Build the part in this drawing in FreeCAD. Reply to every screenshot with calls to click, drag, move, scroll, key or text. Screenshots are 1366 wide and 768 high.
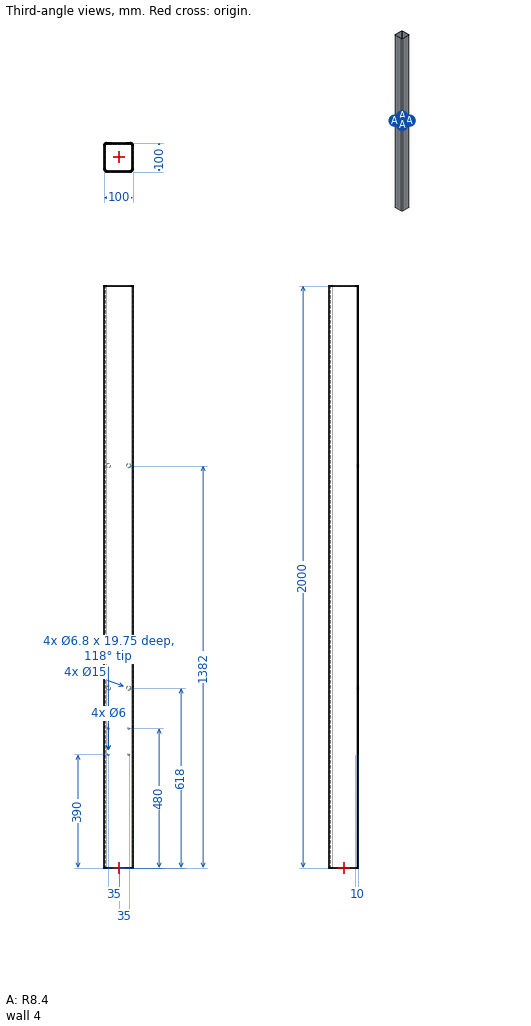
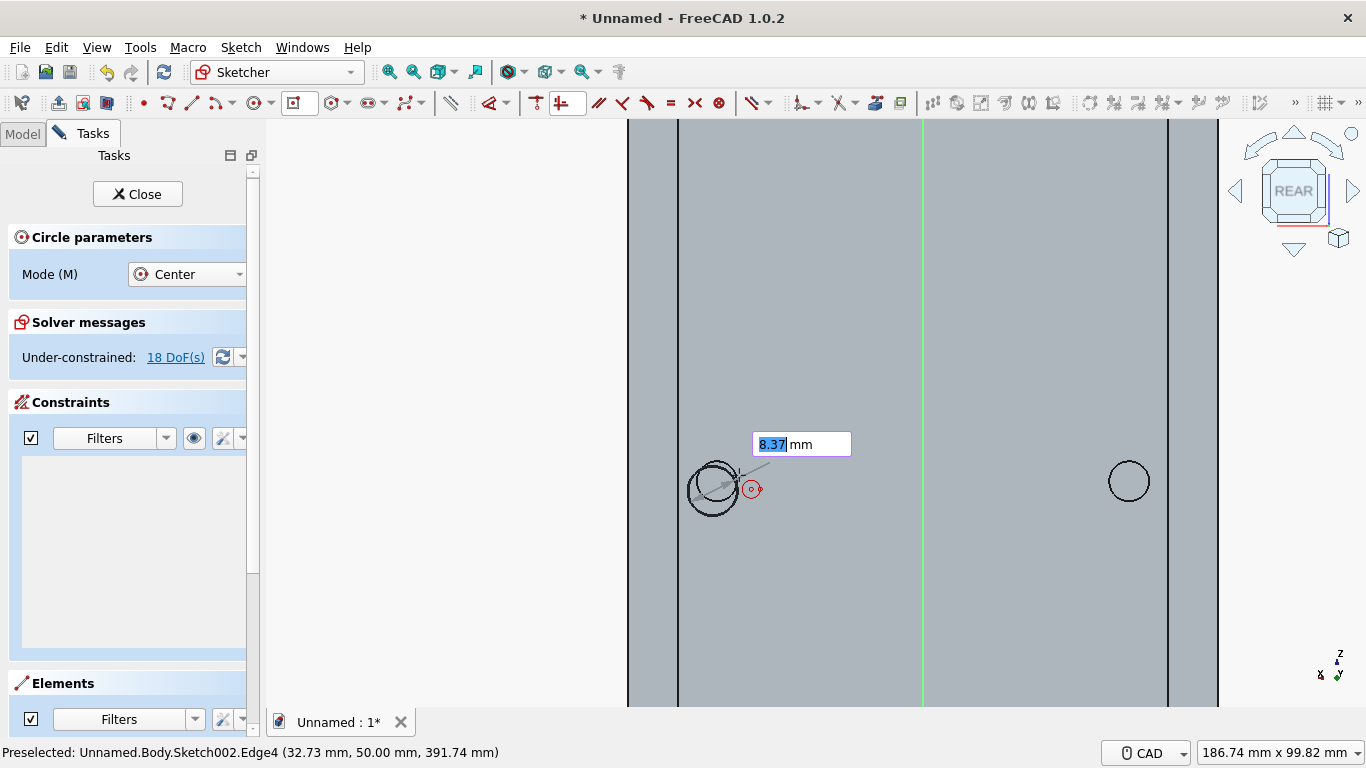
click(729, 469)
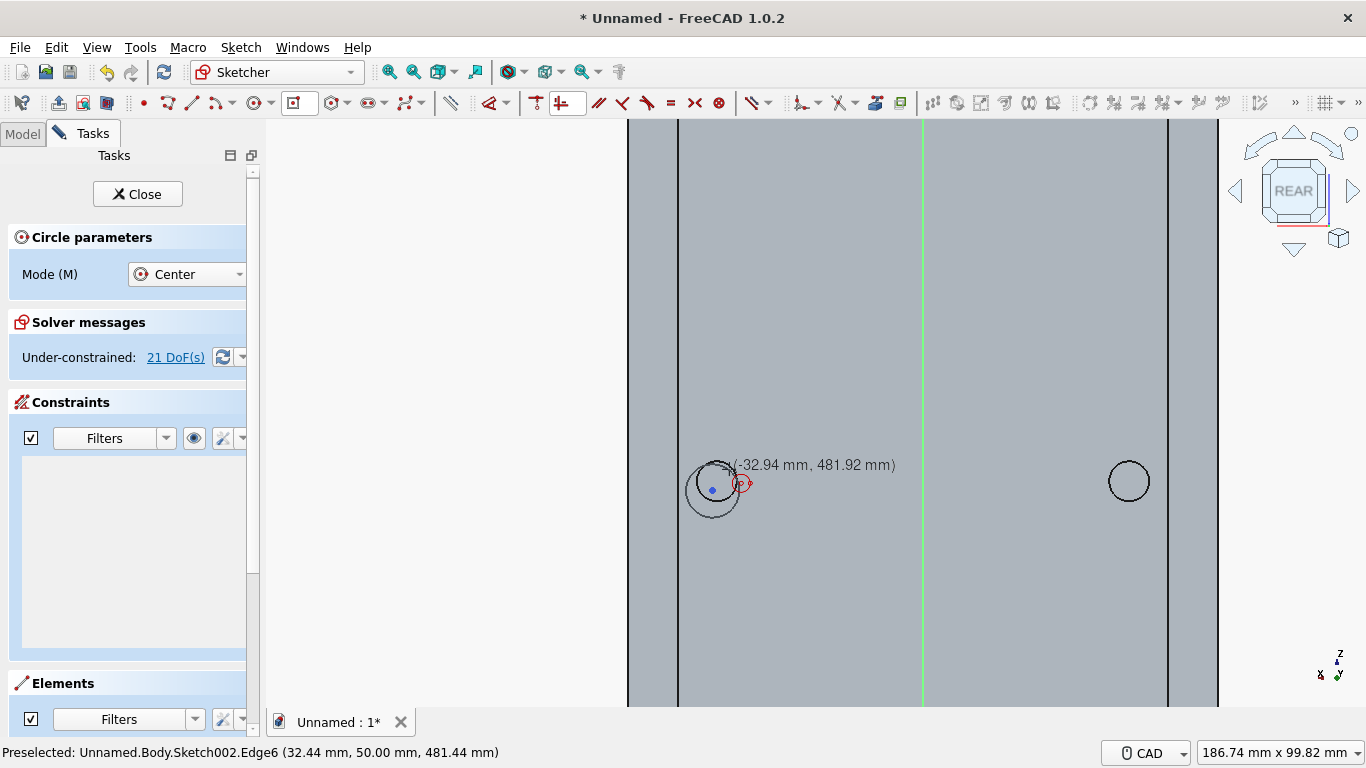
scroll(1129, 481, up, 2)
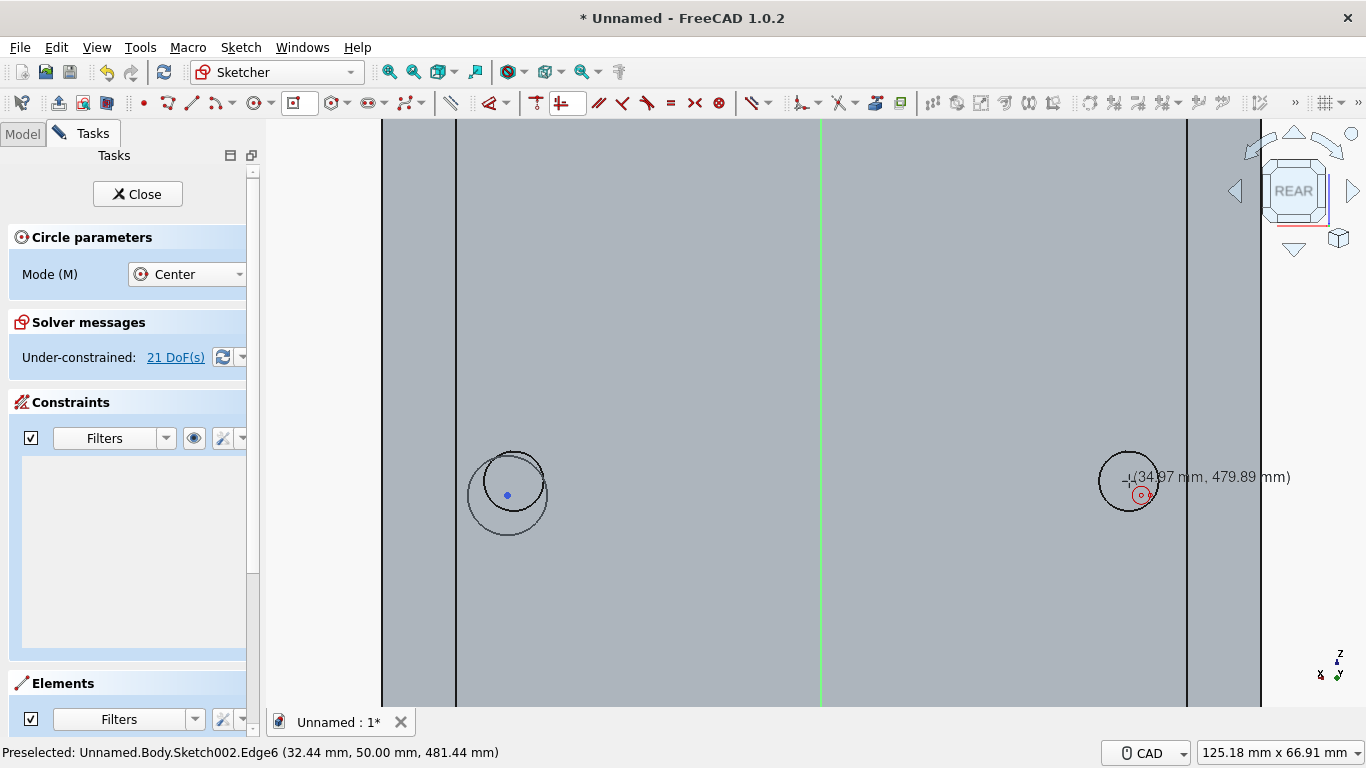
scroll(745, 476, down, 17)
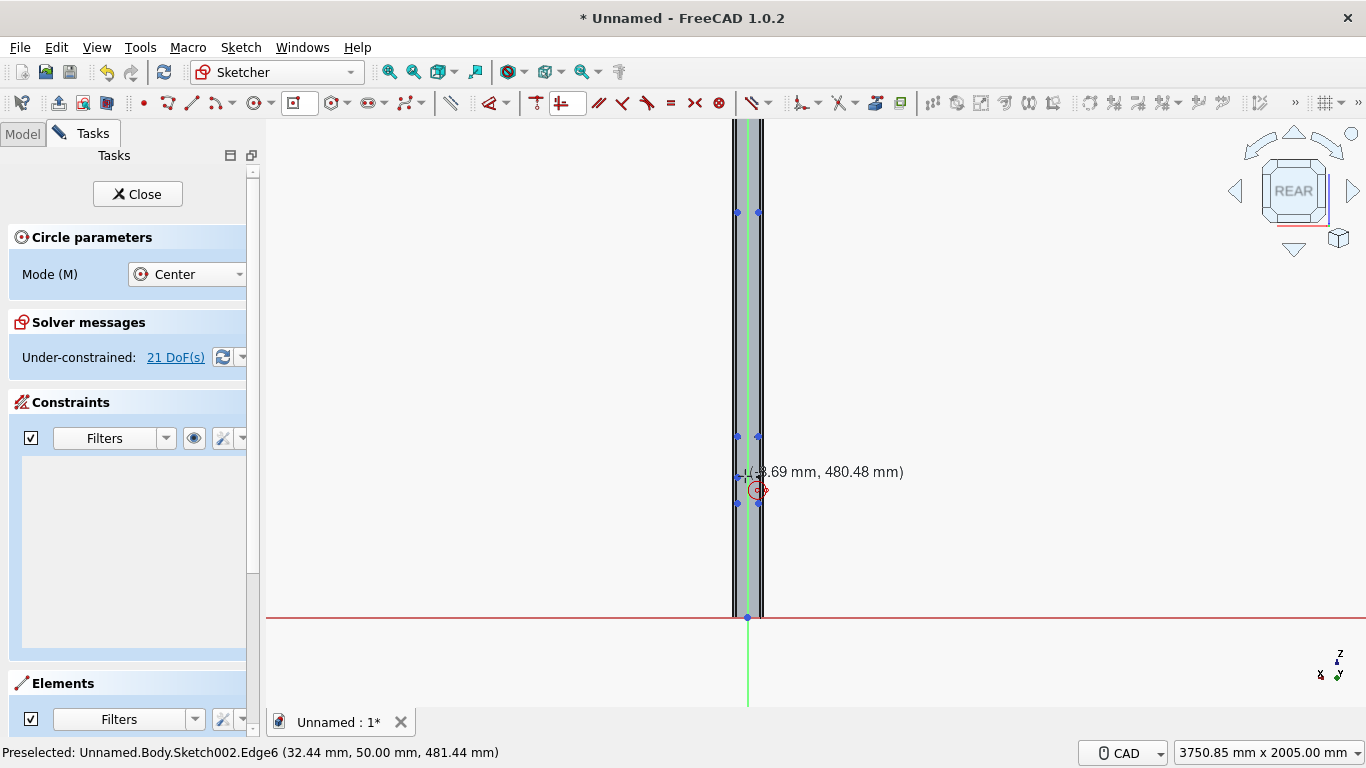
scroll(758, 477, up, 3)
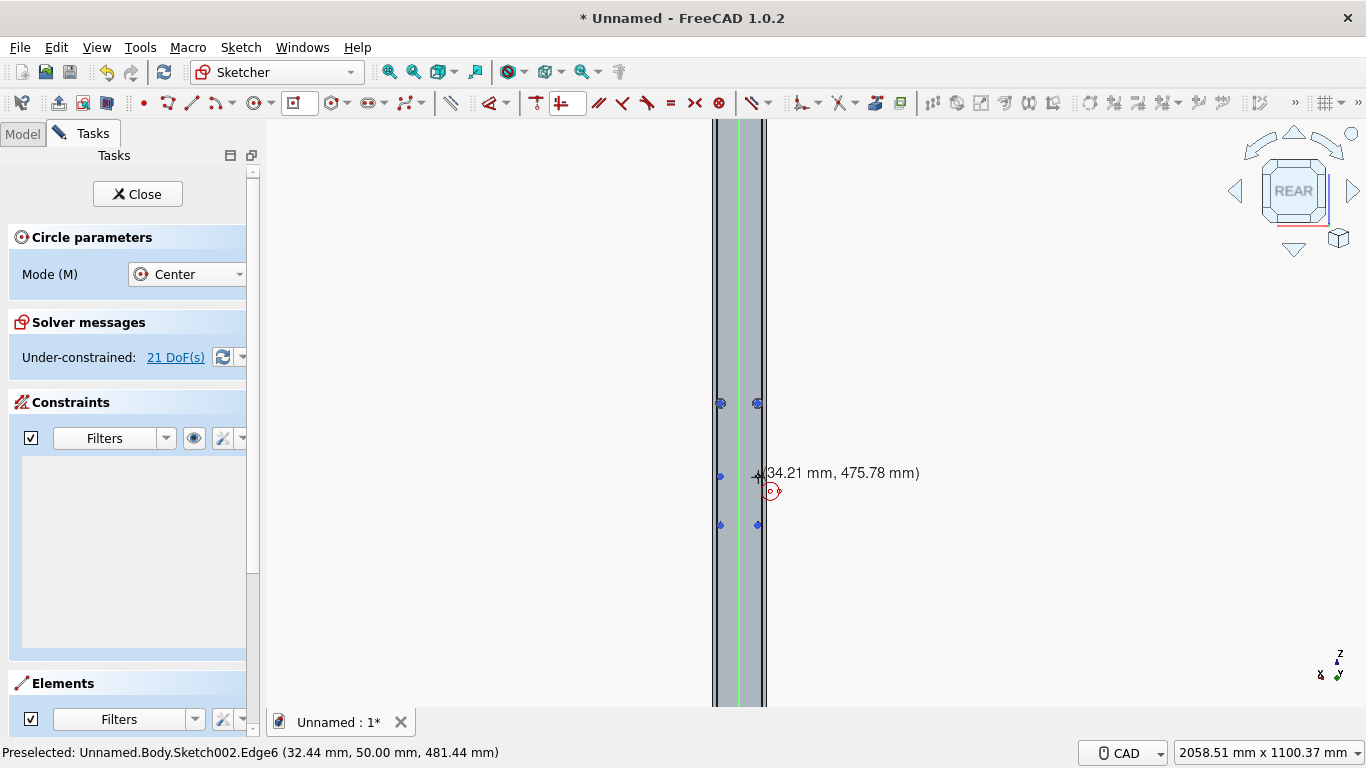
click(758, 476)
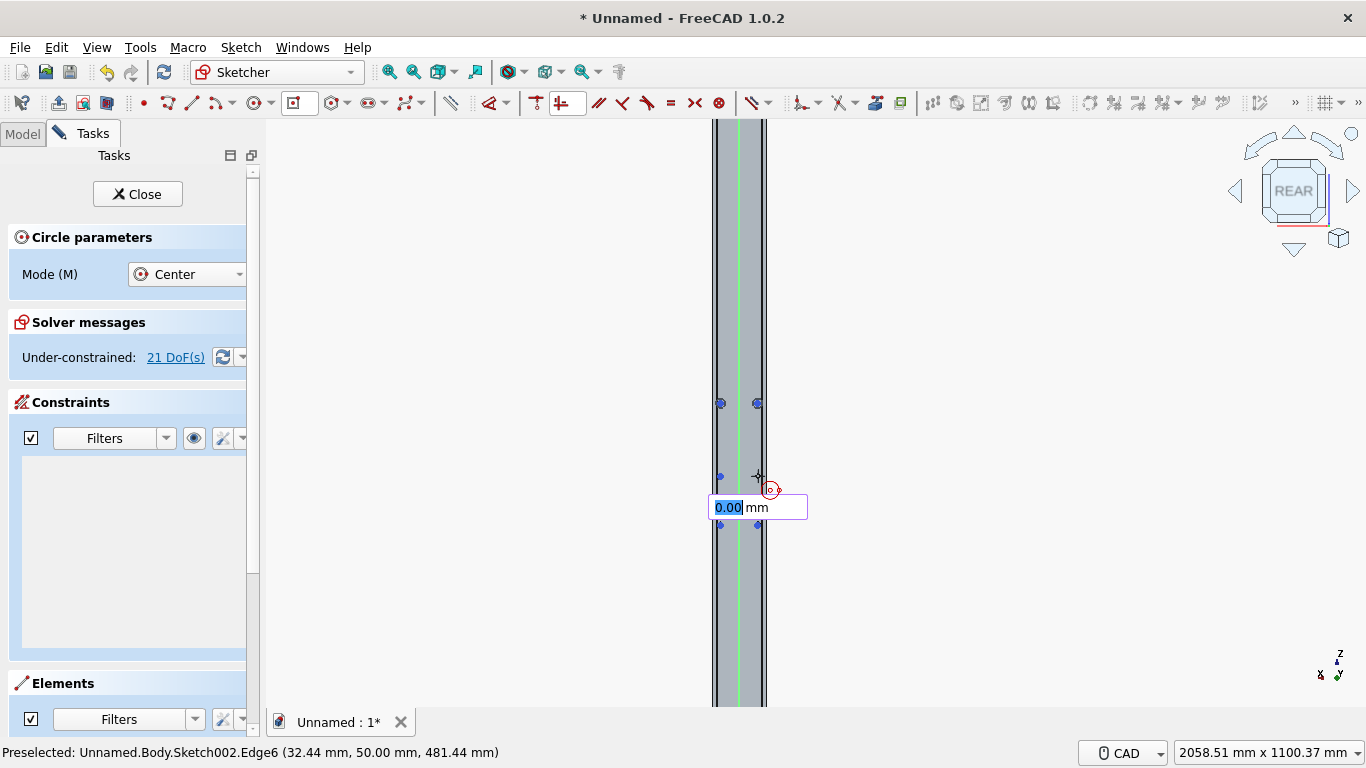
scroll(759, 475, up, 12)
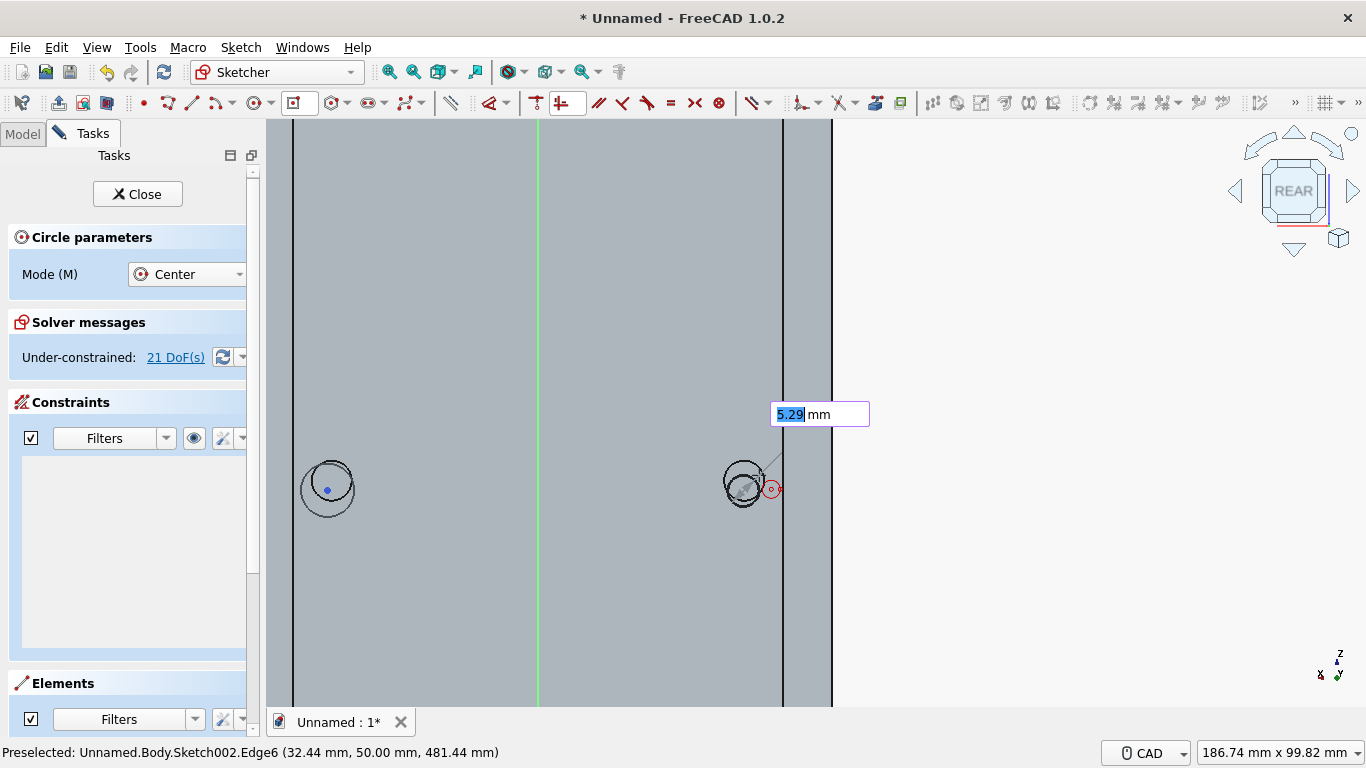
click(757, 468)
key(Escape)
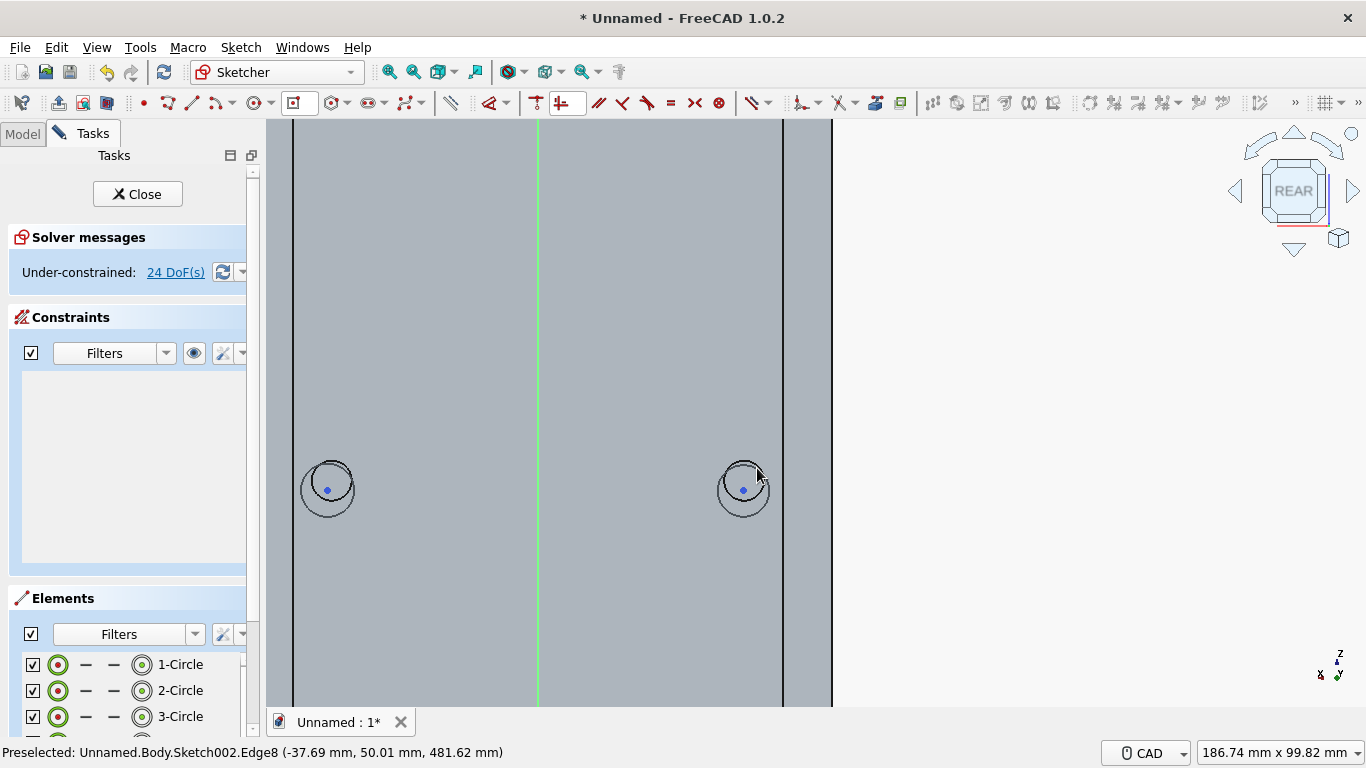
scroll(758, 476, down, 15)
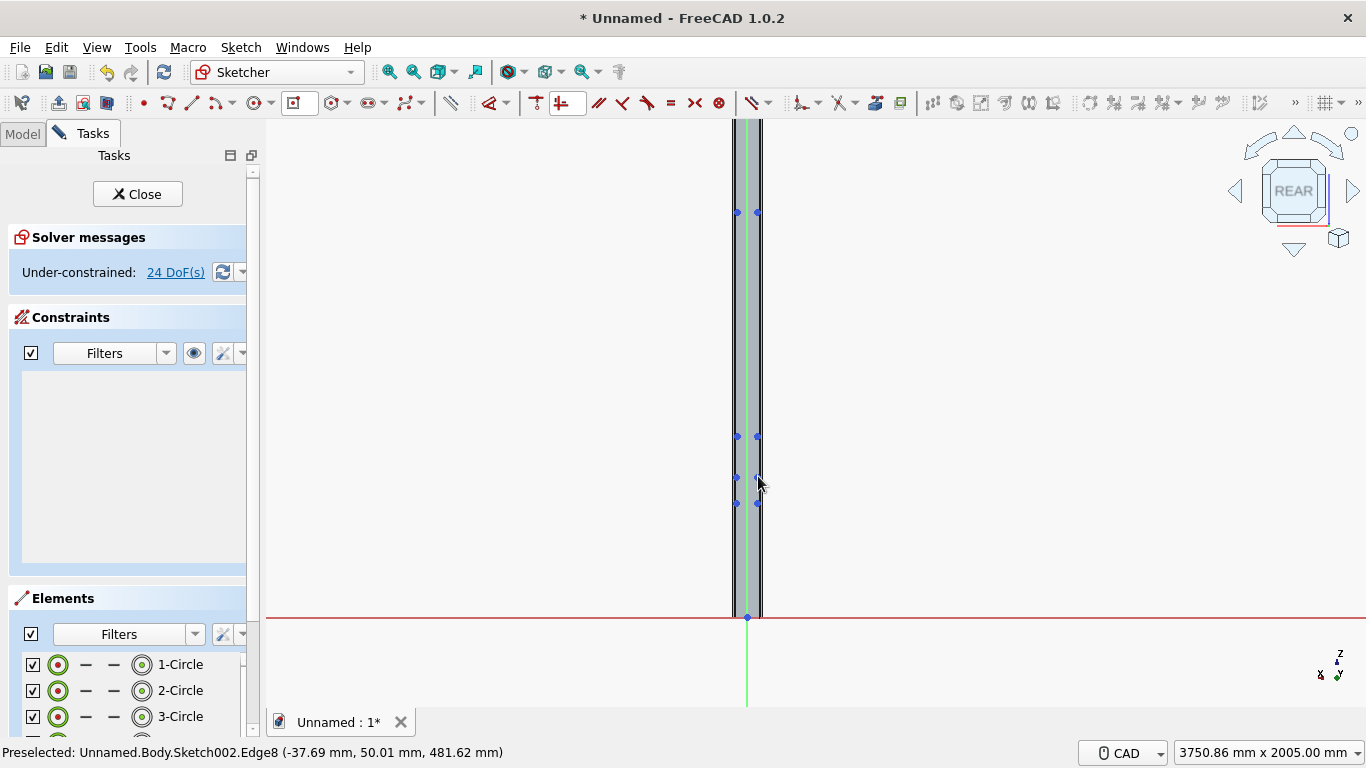
scroll(739, 435, up, 9)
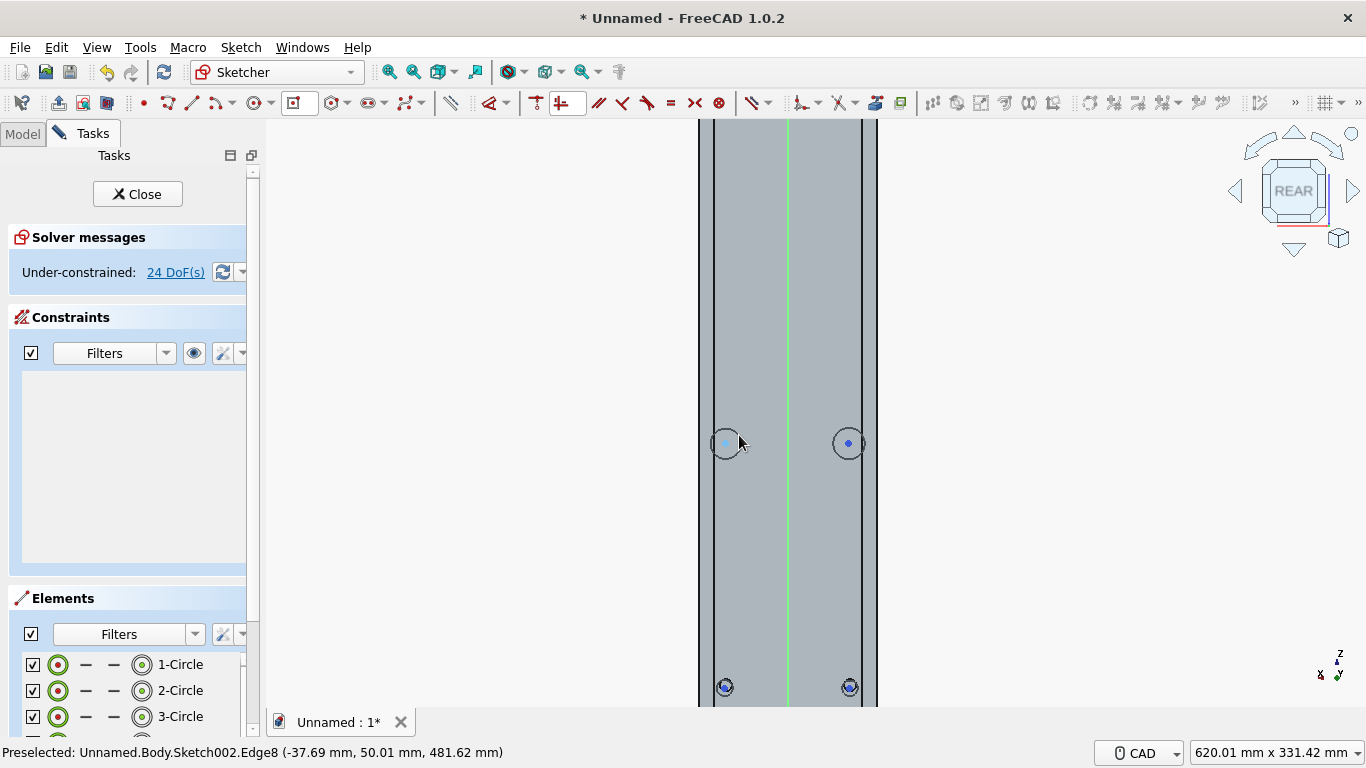
click(737, 433)